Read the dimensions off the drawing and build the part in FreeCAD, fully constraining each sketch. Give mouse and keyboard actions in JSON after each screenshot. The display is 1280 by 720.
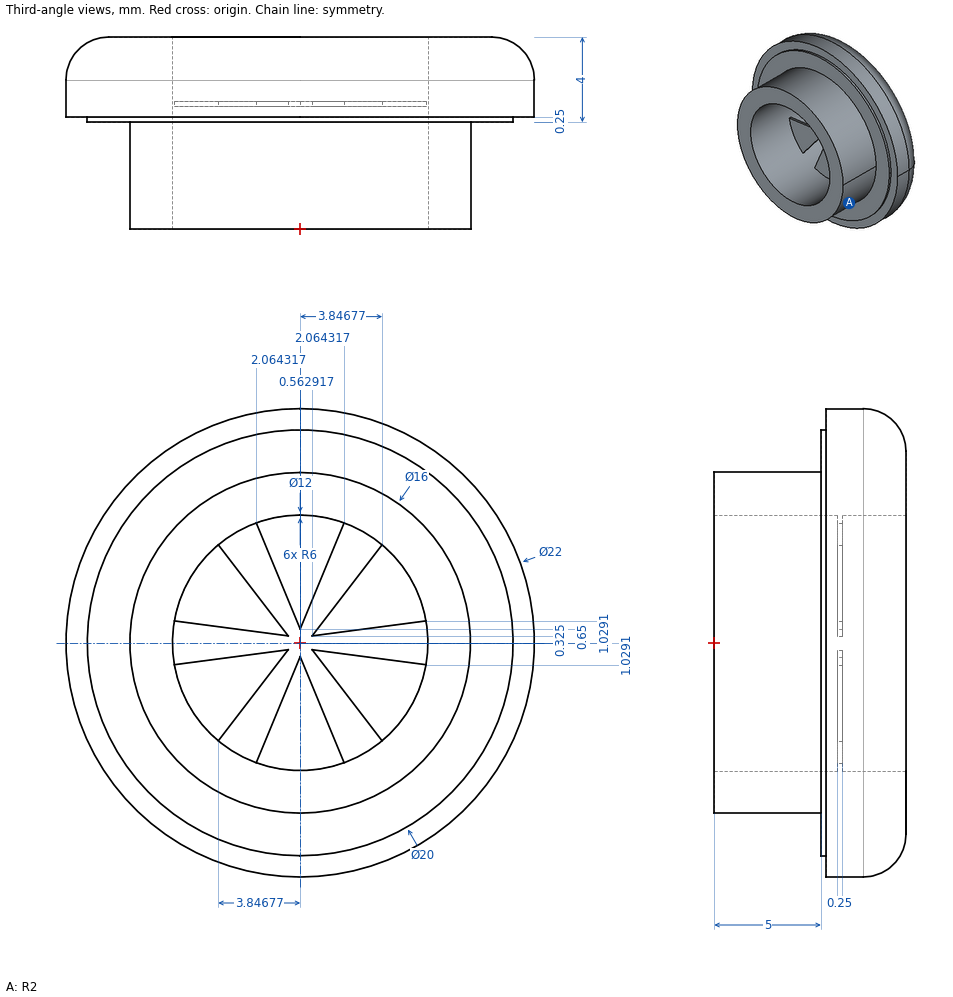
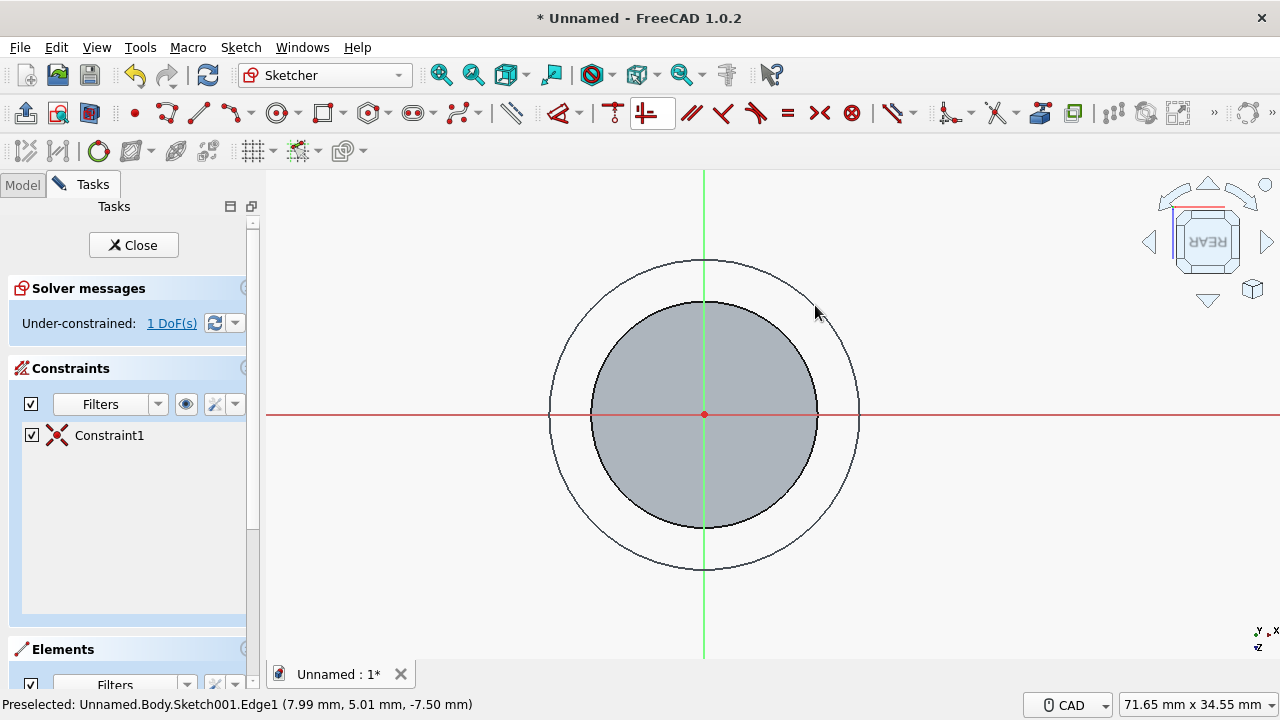
{"action": "key", "text": "d"}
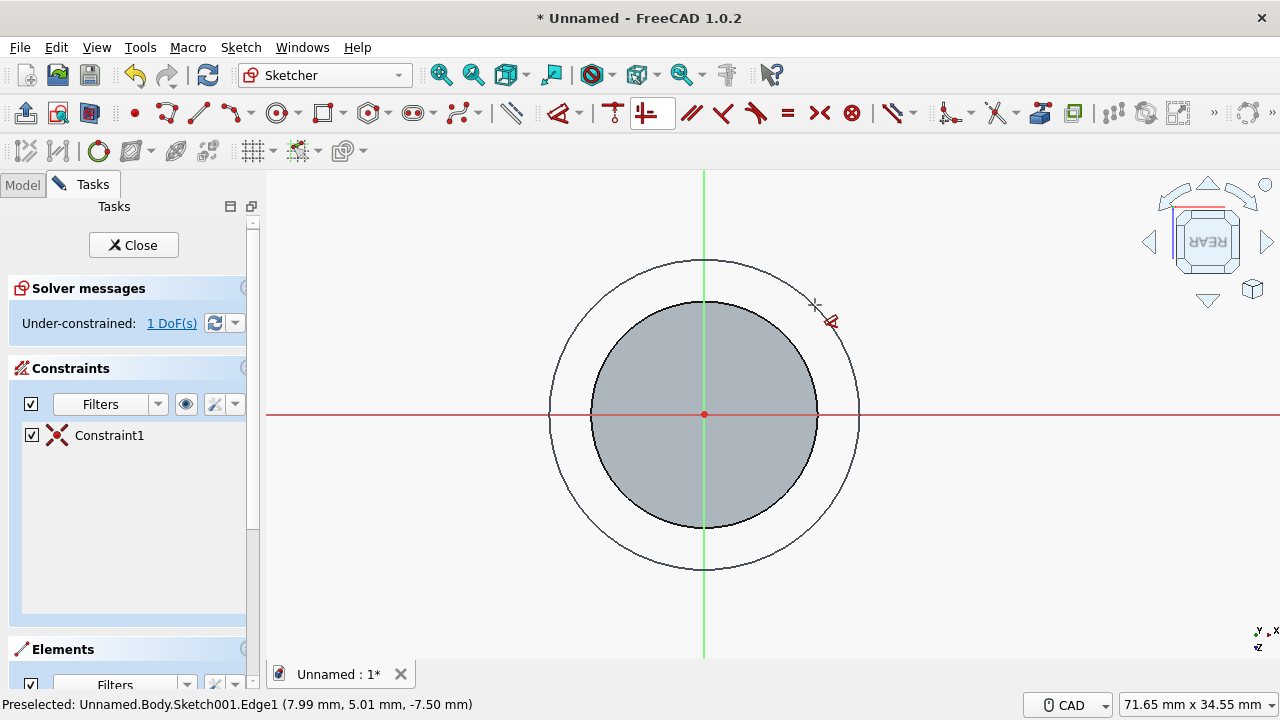
{"action": "left_click", "coordinate": [814, 305]}
{"action": "left_click", "coordinate": [837, 282]}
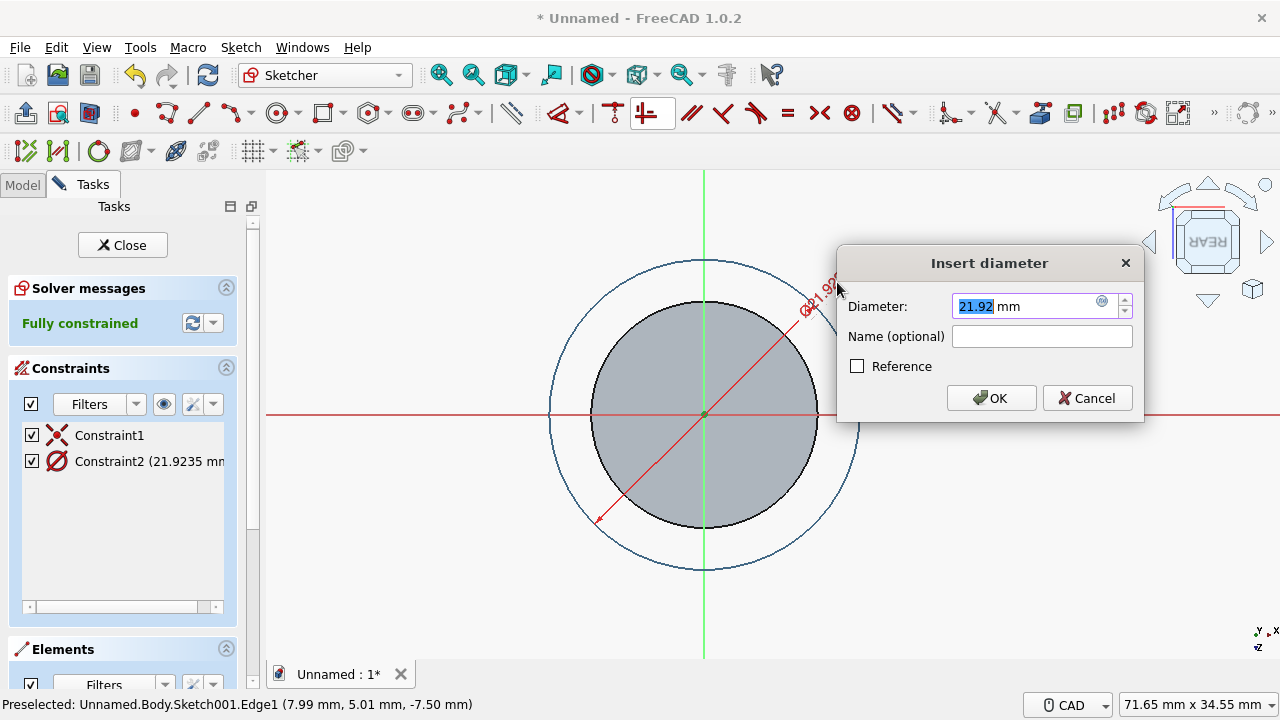
{"action": "type", "text": "22"}
{"action": "key", "text": "Return"}
{"action": "key", "text": "Escape"}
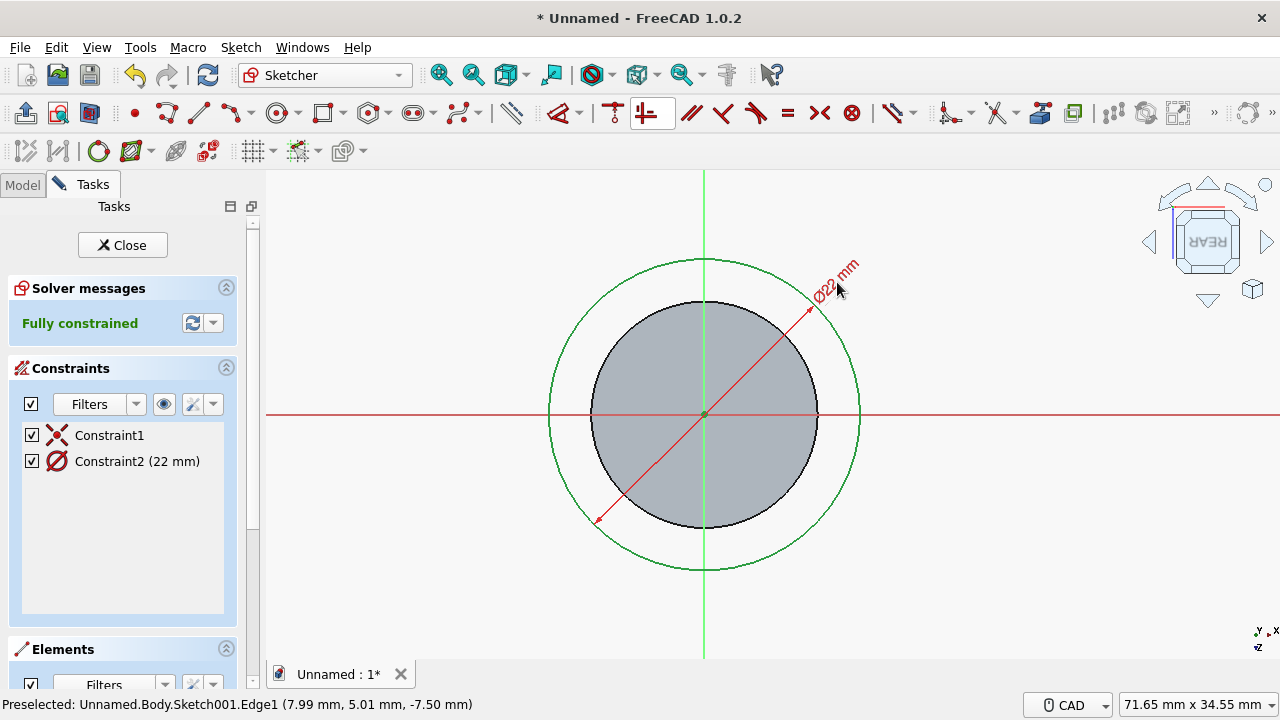
{"action": "left_click", "coordinate": [123, 245]}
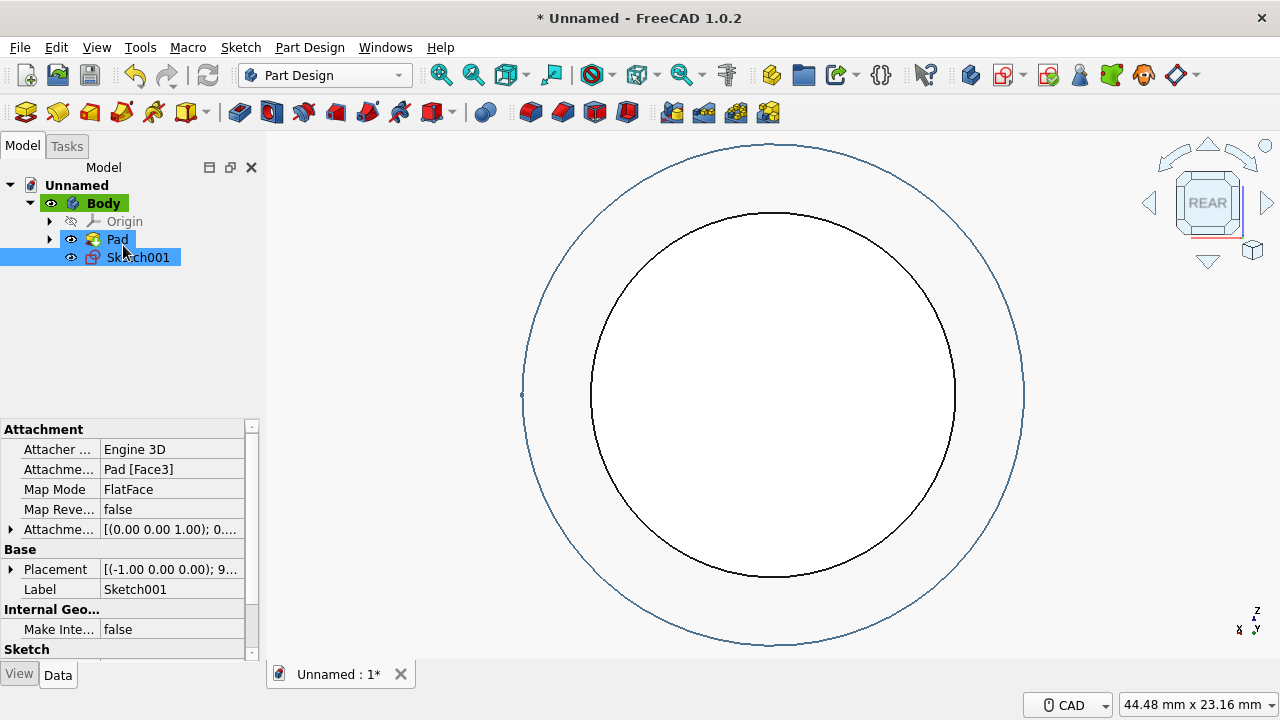
{"action": "left_click", "coordinate": [26, 112]}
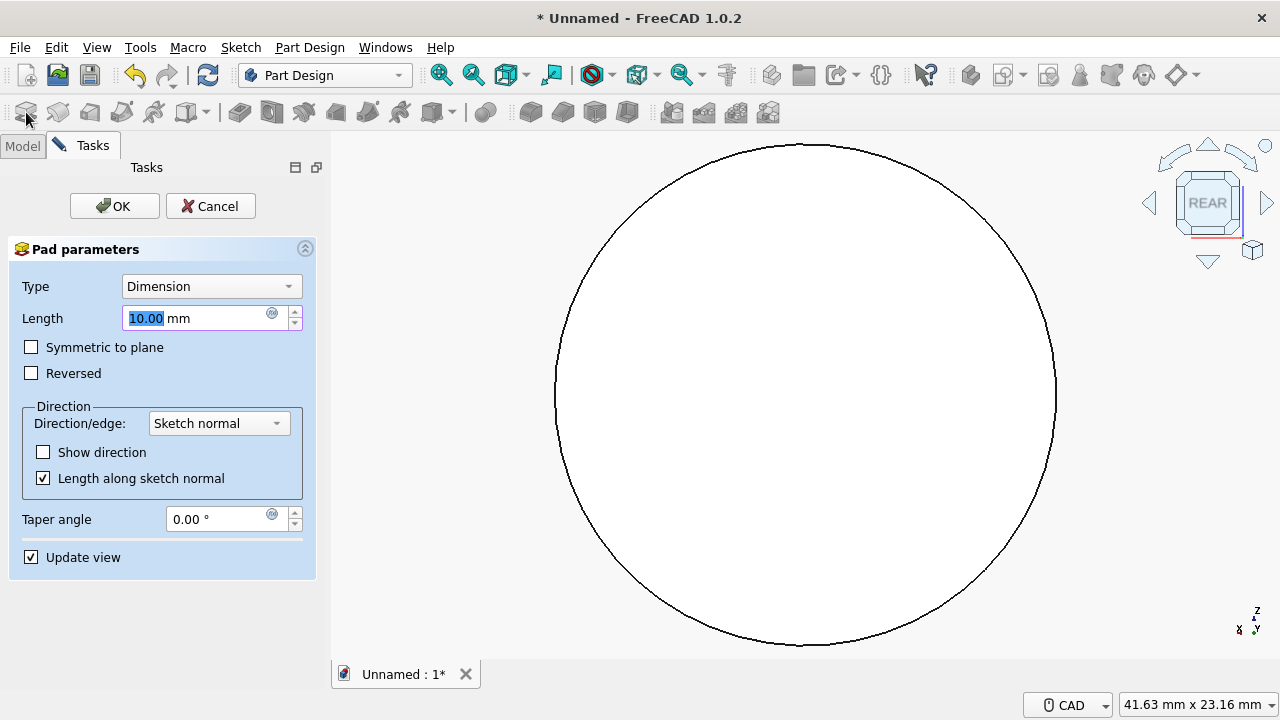
{"action": "type", "text": "4"}
{"action": "key", "text": "Tab"}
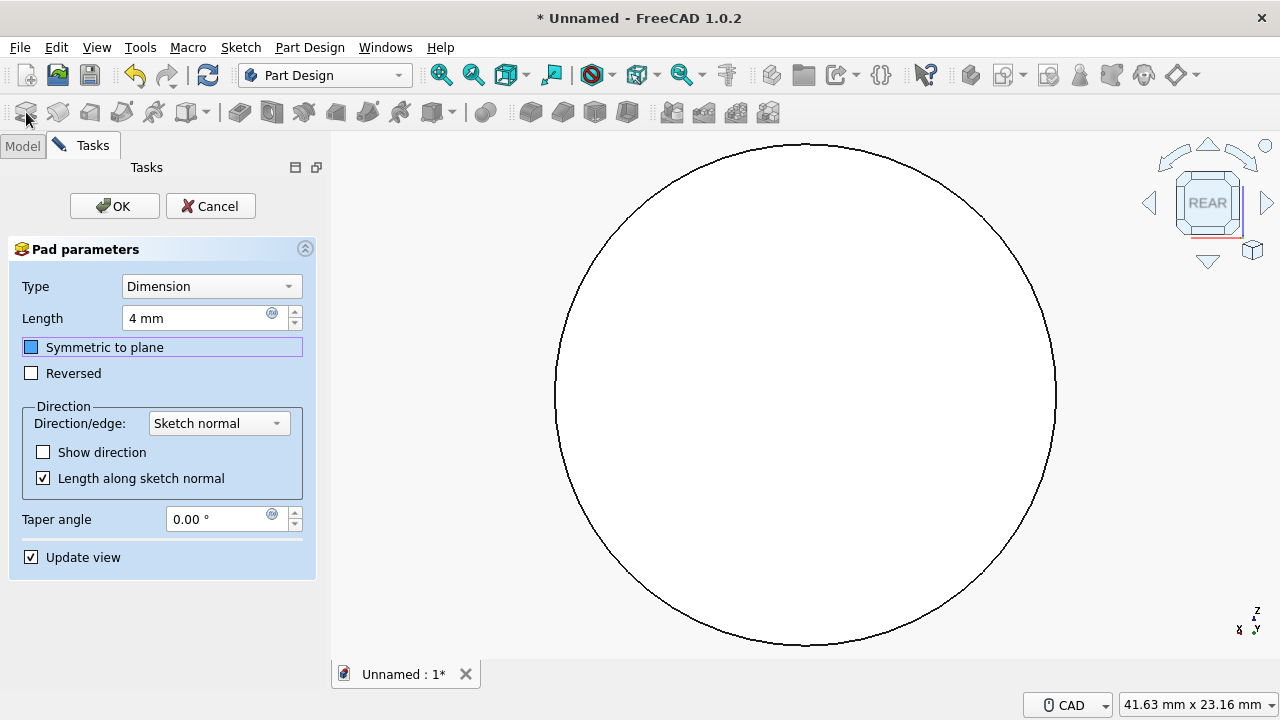
{"action": "left_click", "coordinate": [115, 206]}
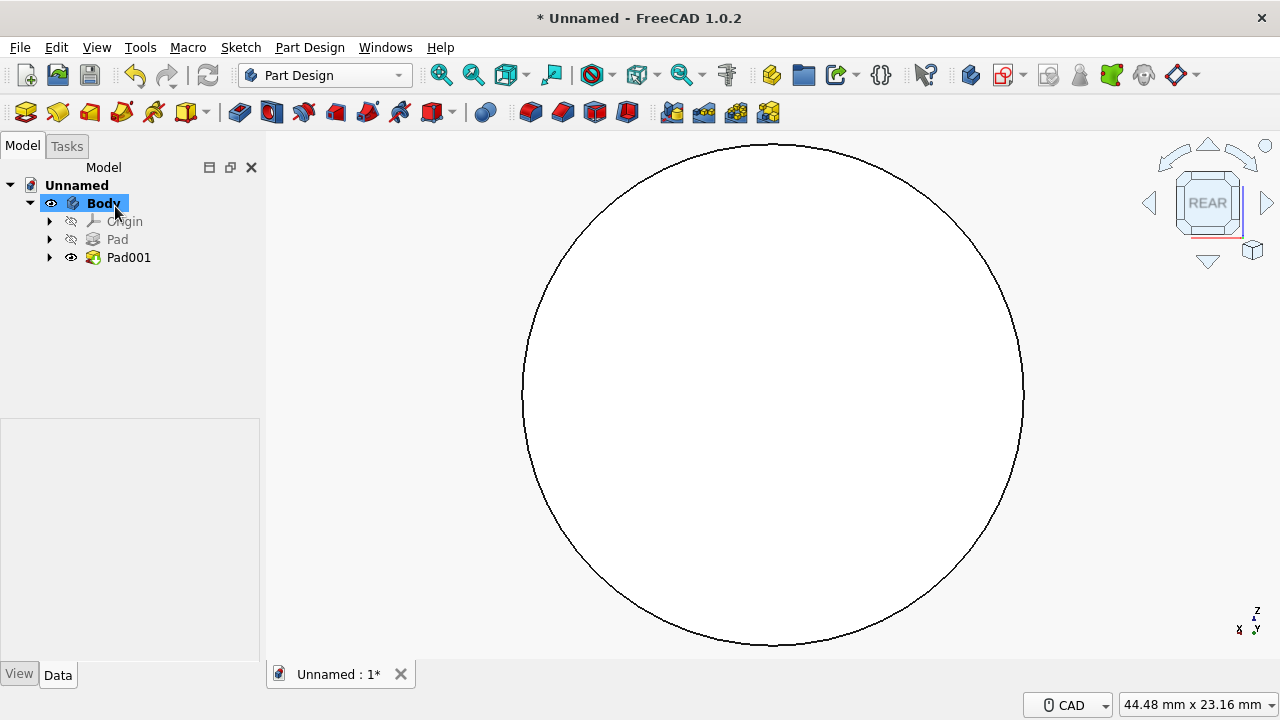
{"action": "left_click", "coordinate": [773, 394]}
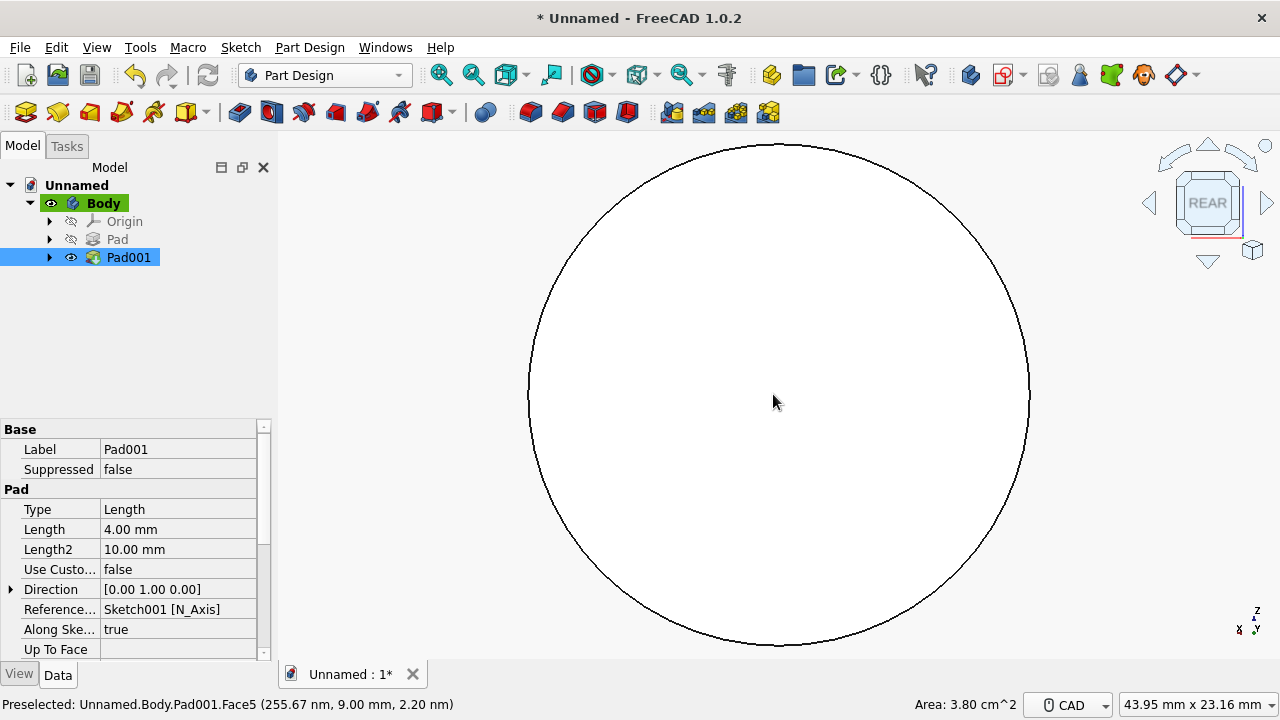
{"action": "left_click", "coordinate": [1004, 76]}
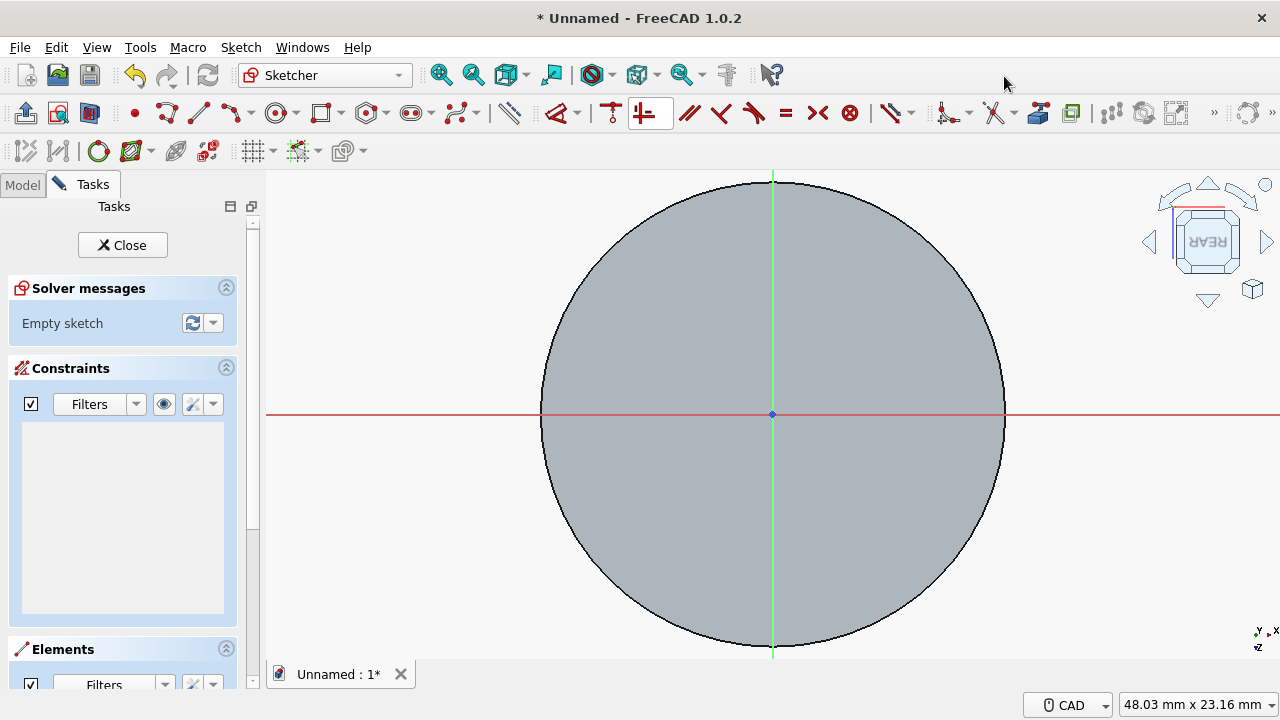
{"action": "left_click", "coordinate": [276, 114]}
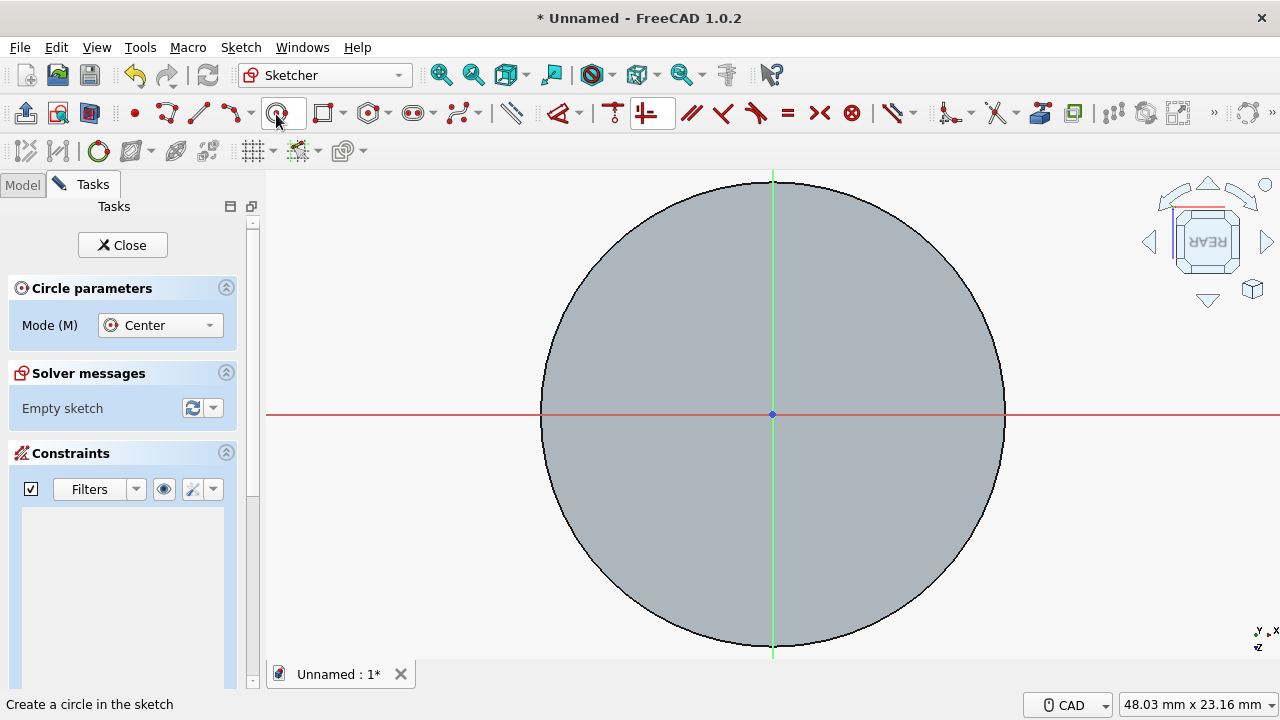
{"action": "left_click", "coordinate": [773, 414]}
{"action": "left_click", "coordinate": [863, 325]}
{"action": "key", "text": "Escape"}